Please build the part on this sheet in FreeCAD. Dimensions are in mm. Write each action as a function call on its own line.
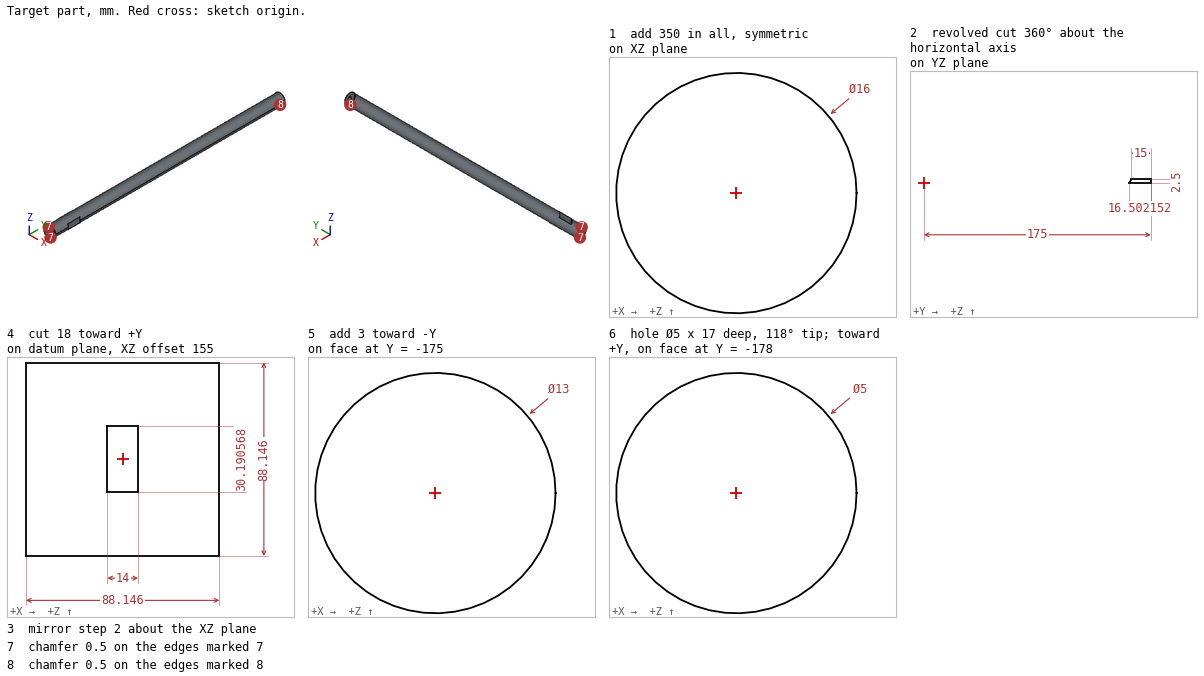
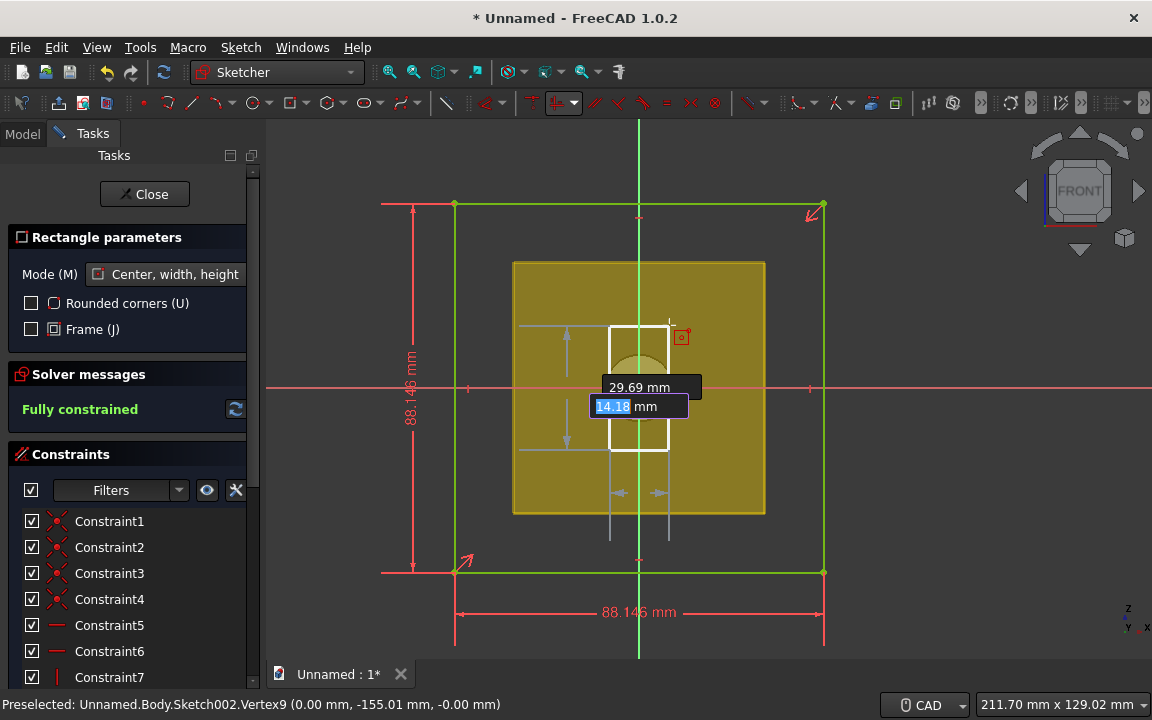
text(14)
key(Tab)
text(30.190568)
key(Return)
key(Escape)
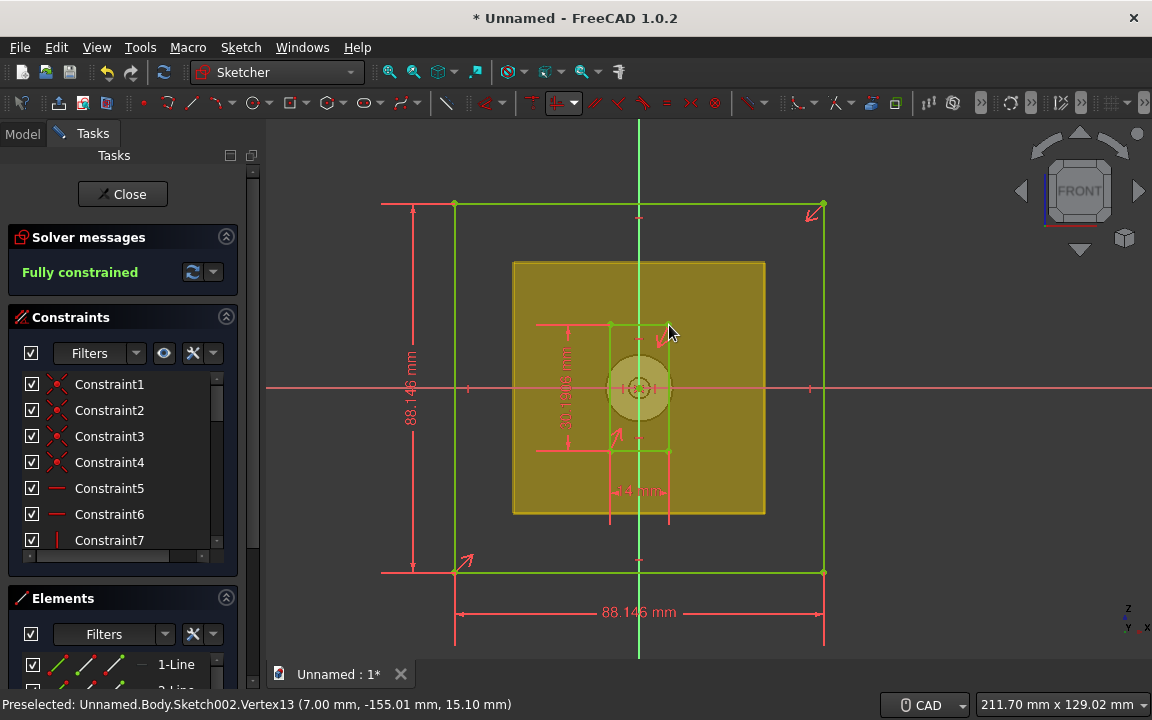
click(123, 194)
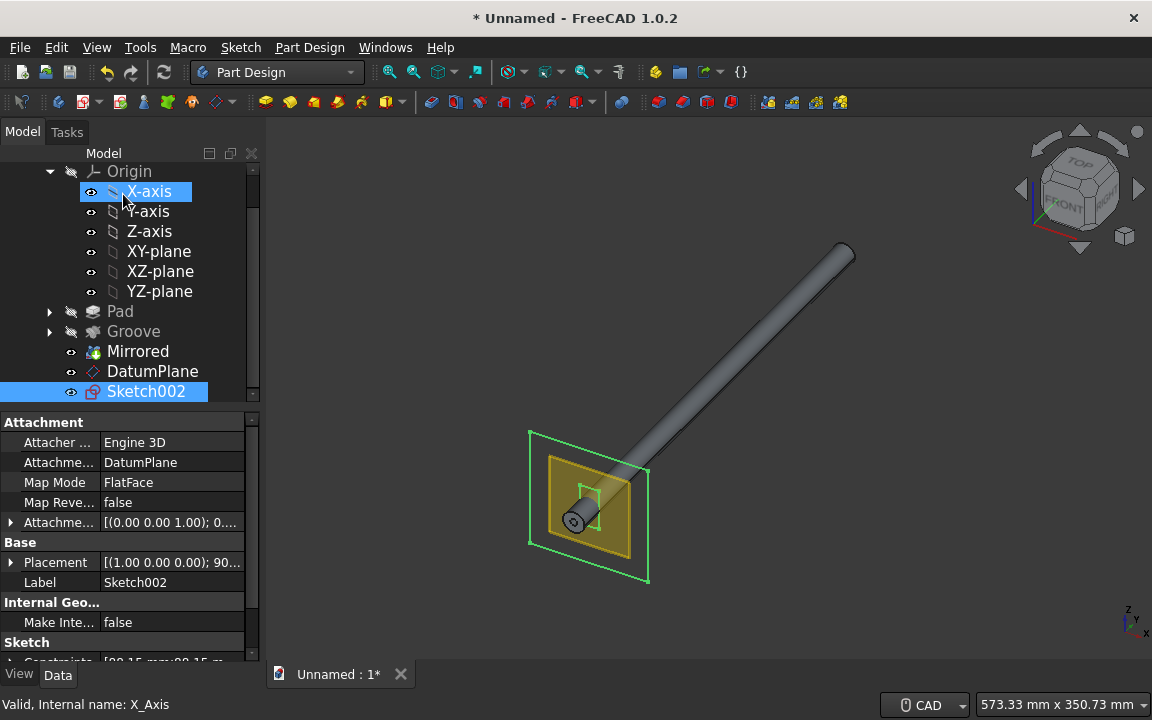
click(432, 102)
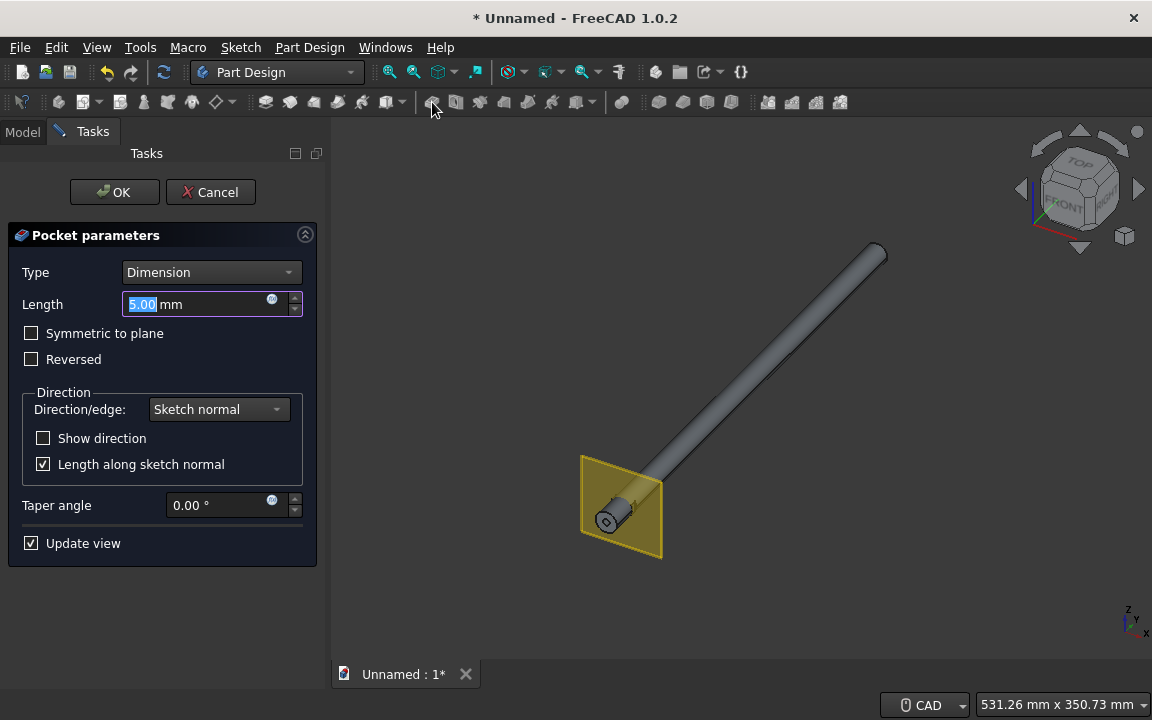
text(18)
key(Tab)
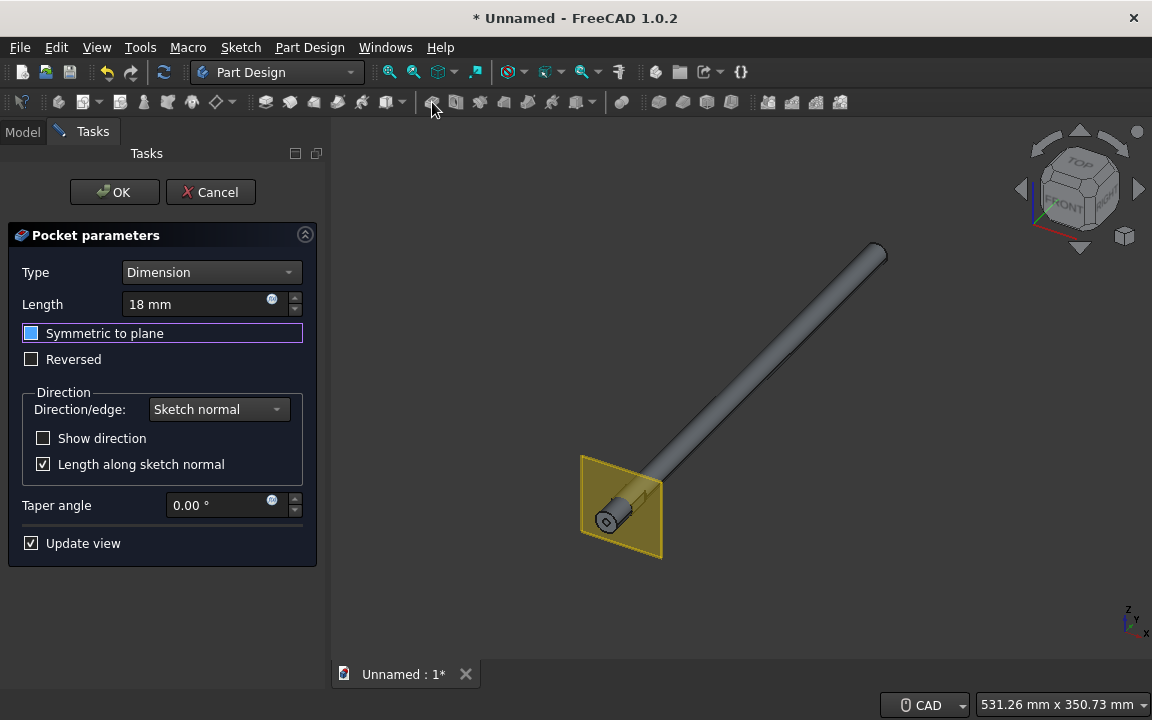
click(115, 192)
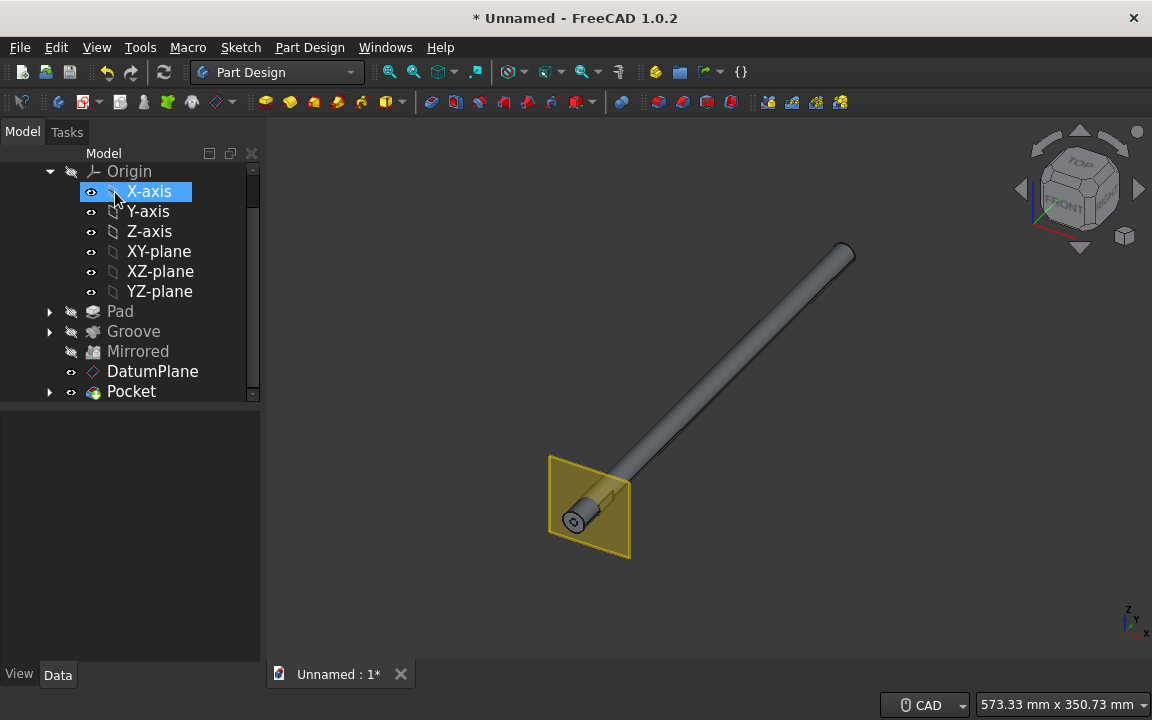
click(116, 372)
key(space)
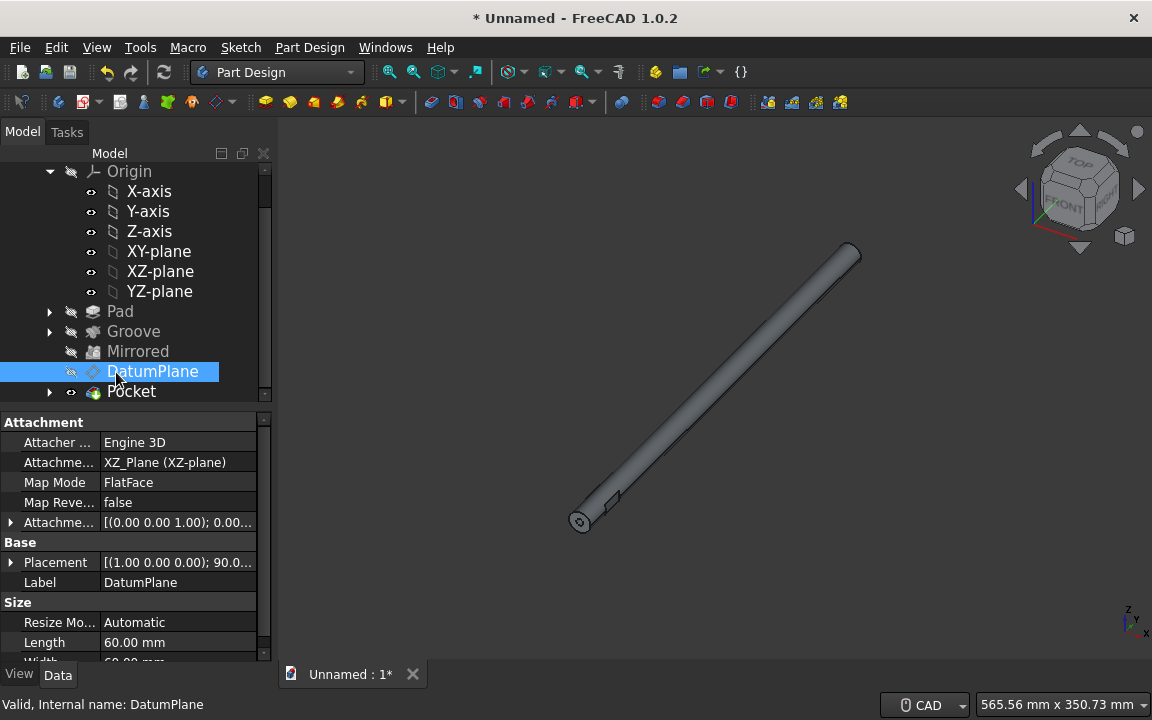
scroll(583, 517, up, 6)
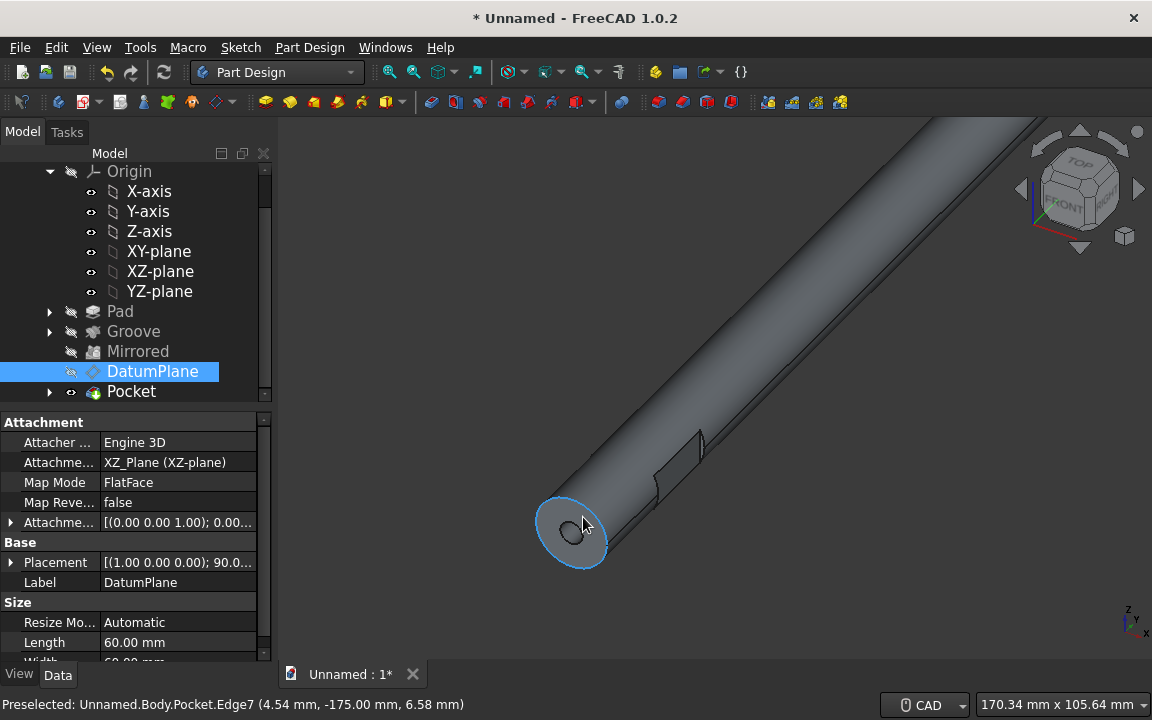
click(582, 516)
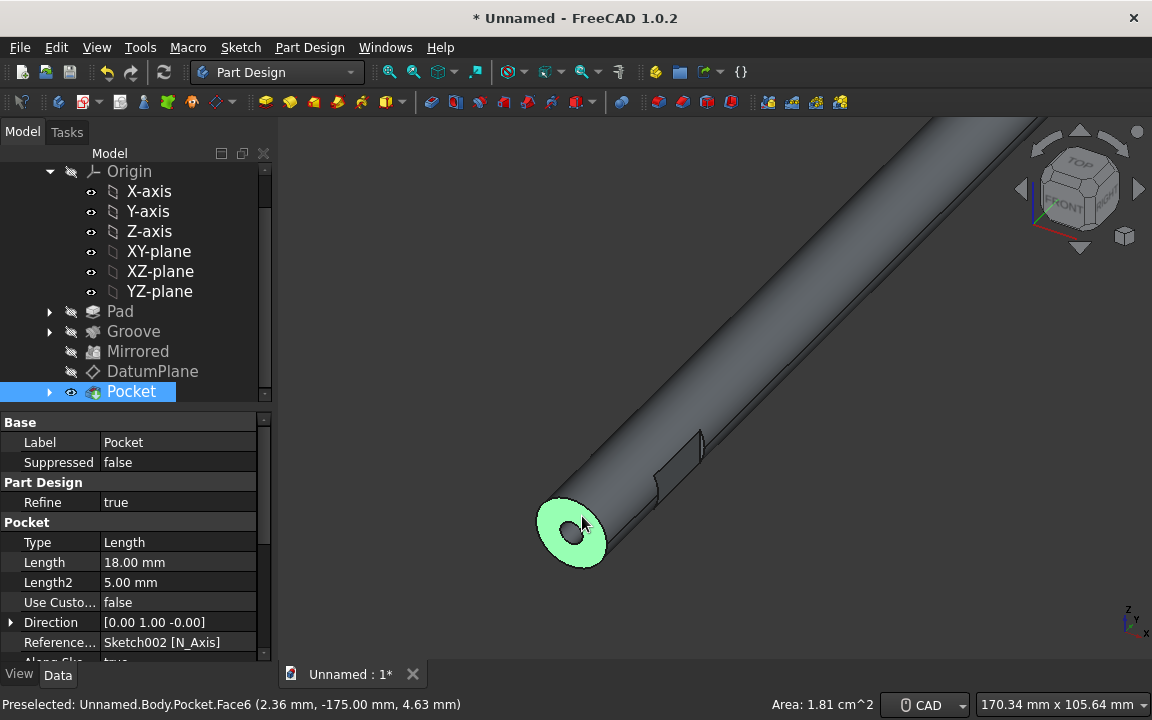
click(84, 102)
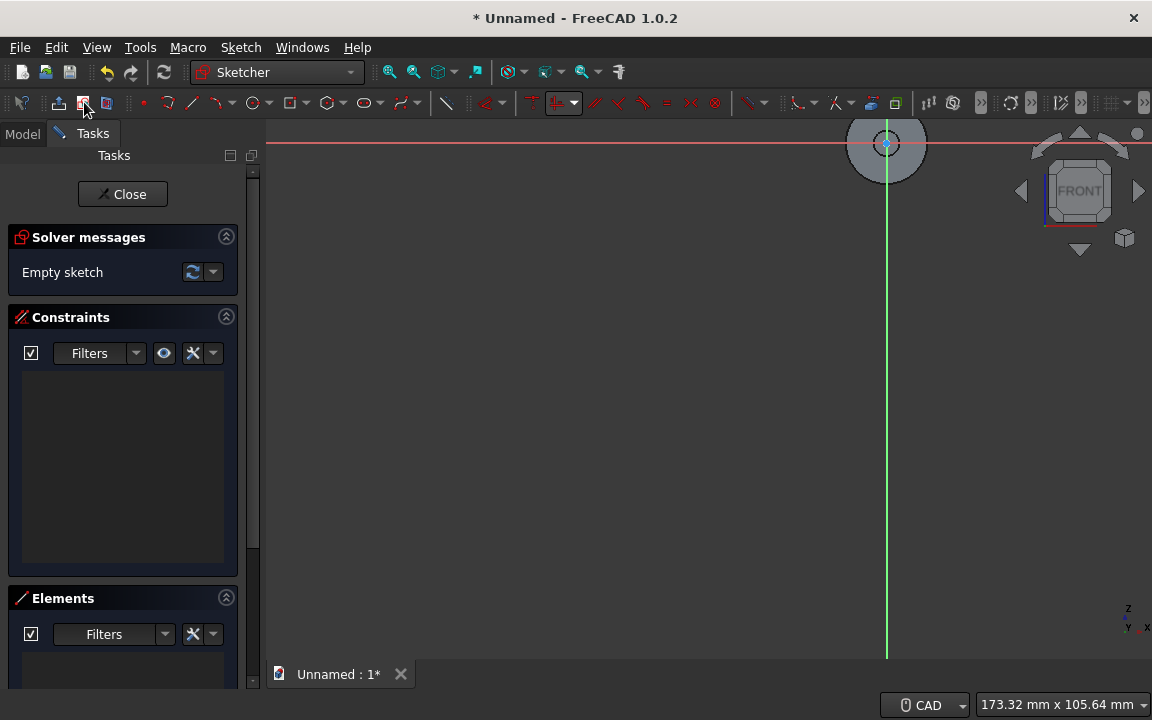
scroll(640, 389, down, 5)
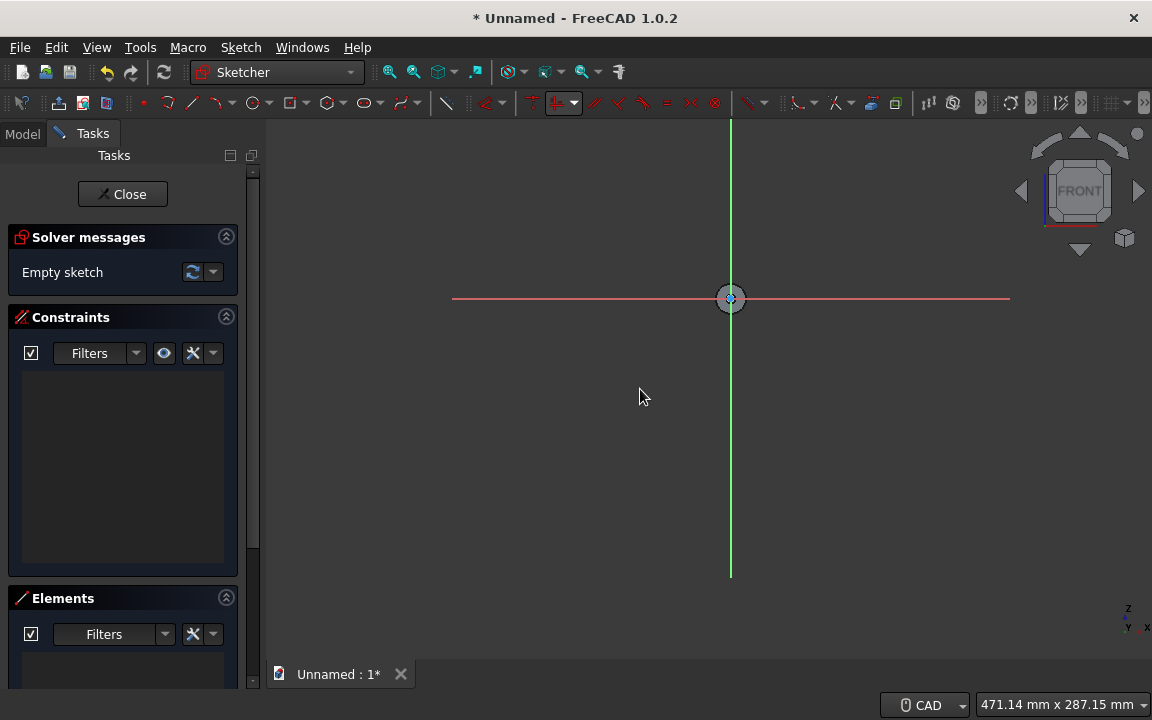
scroll(738, 292, up, 13)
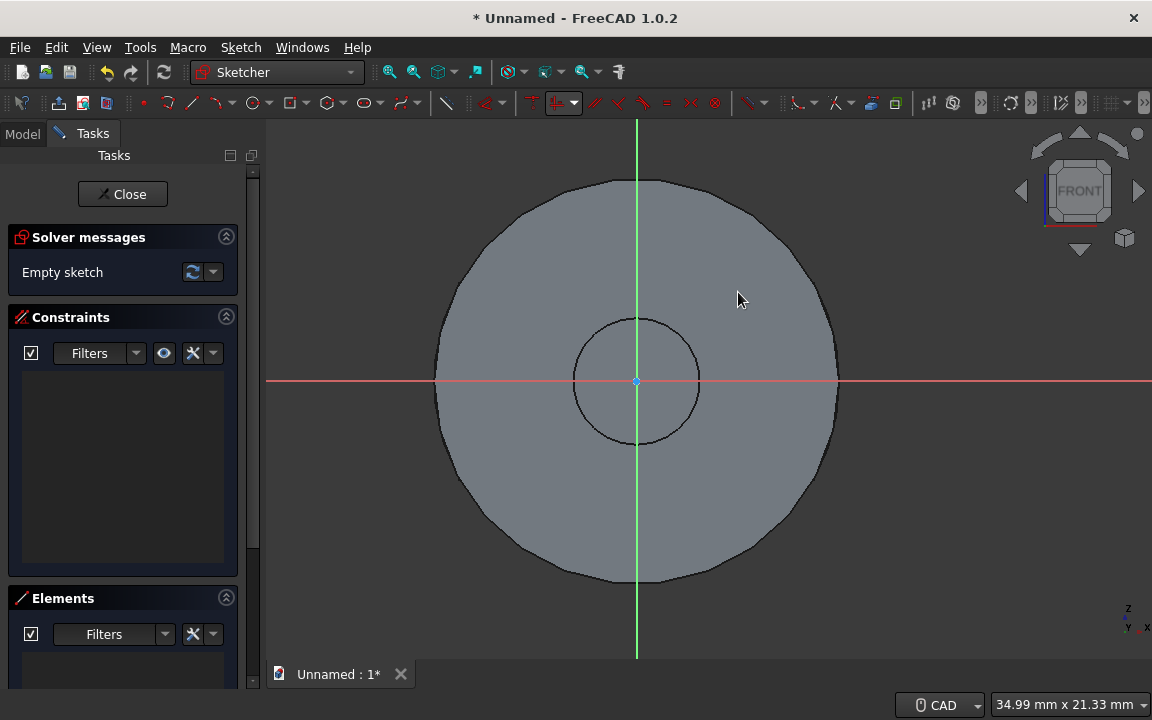
click(254, 104)